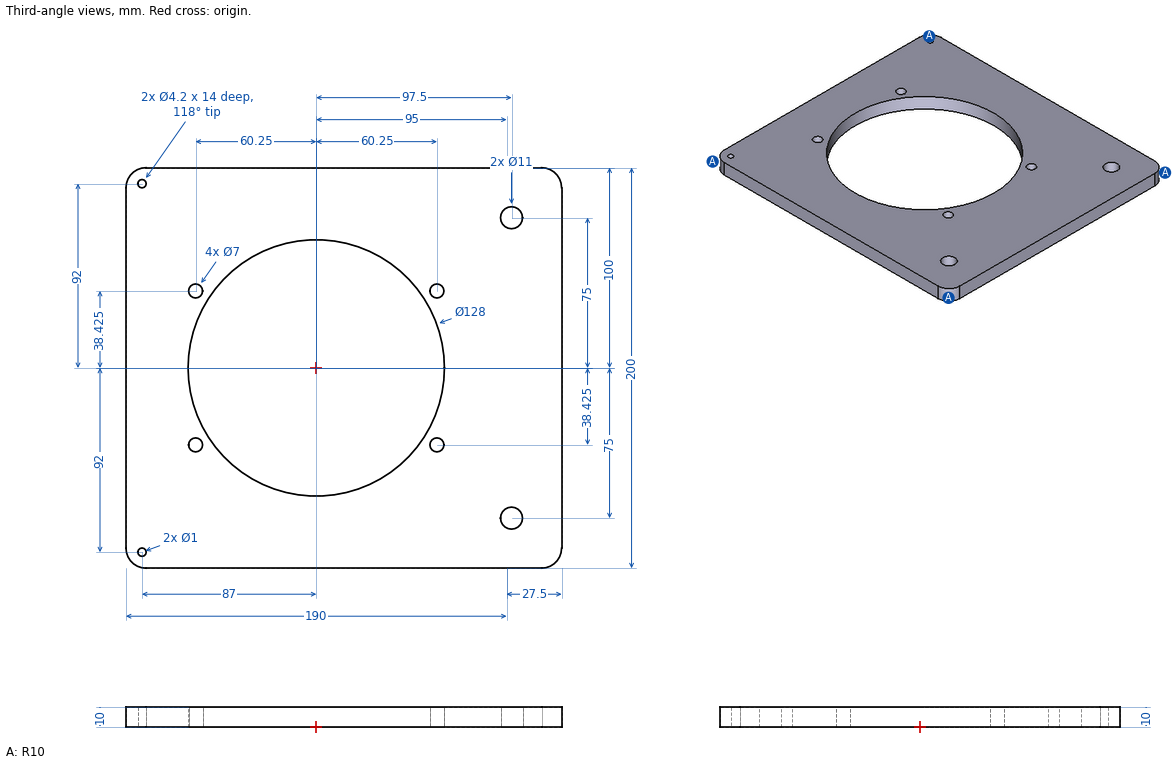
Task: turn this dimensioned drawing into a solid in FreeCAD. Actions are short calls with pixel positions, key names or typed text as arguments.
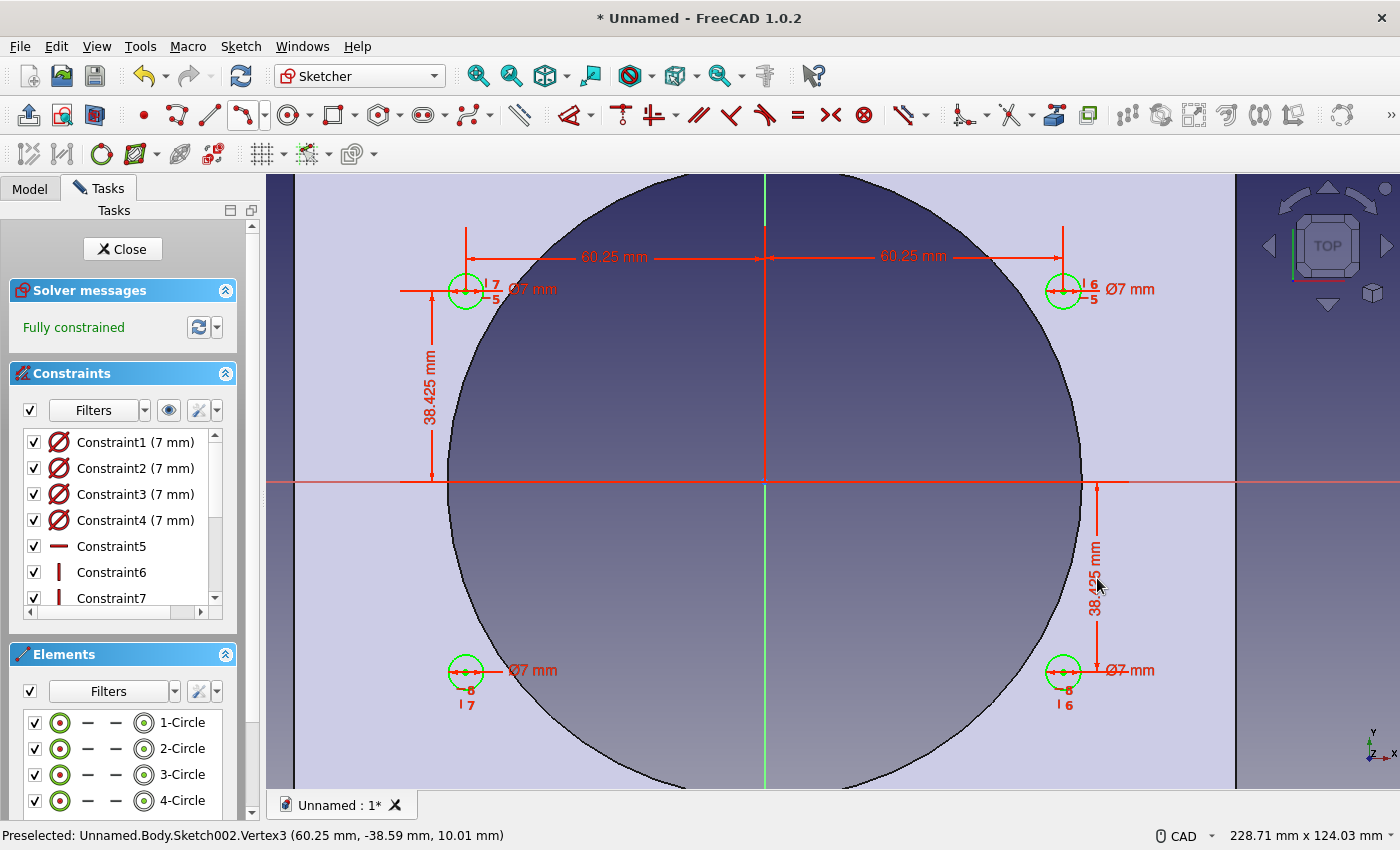
click(123, 249)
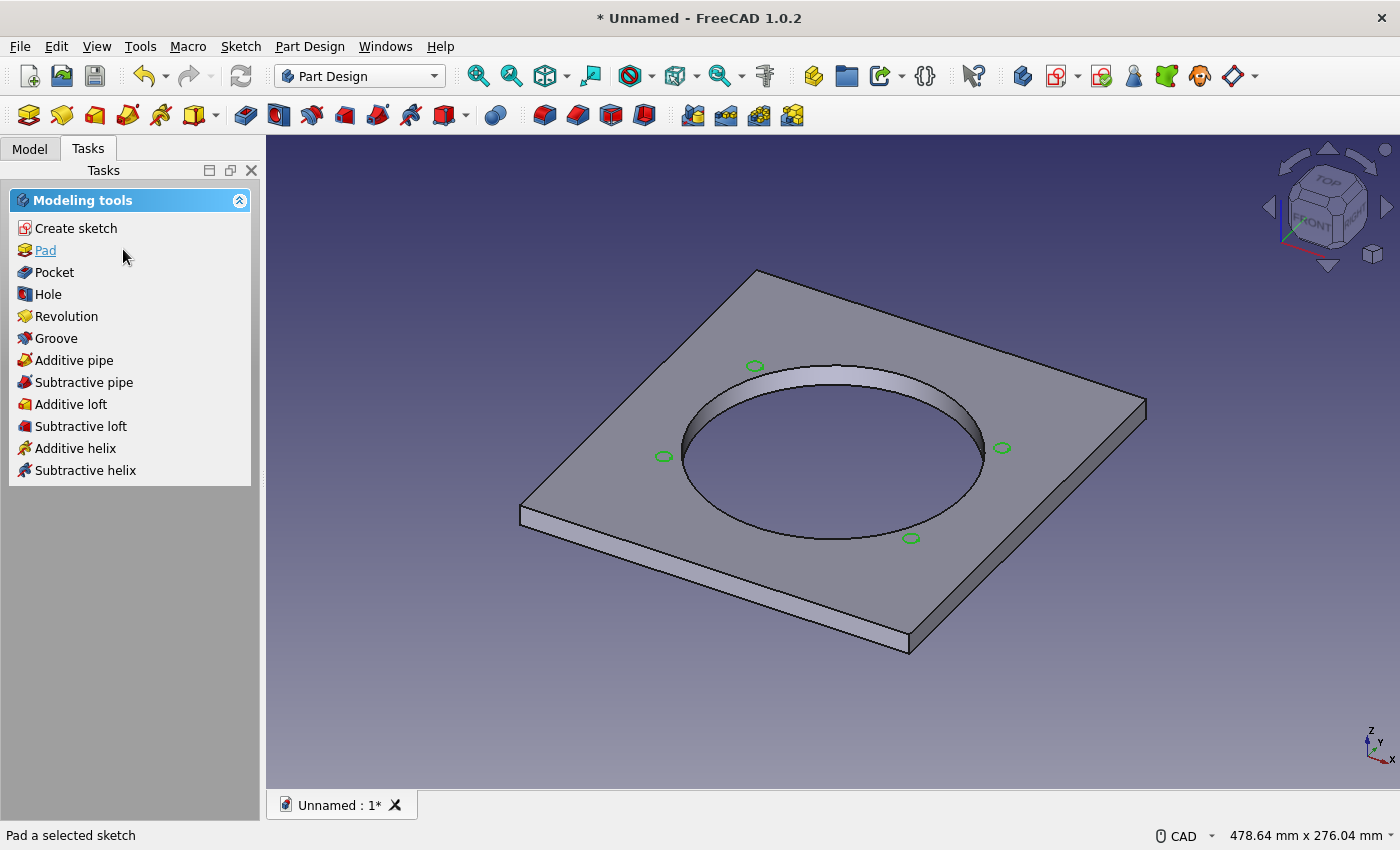
click(246, 116)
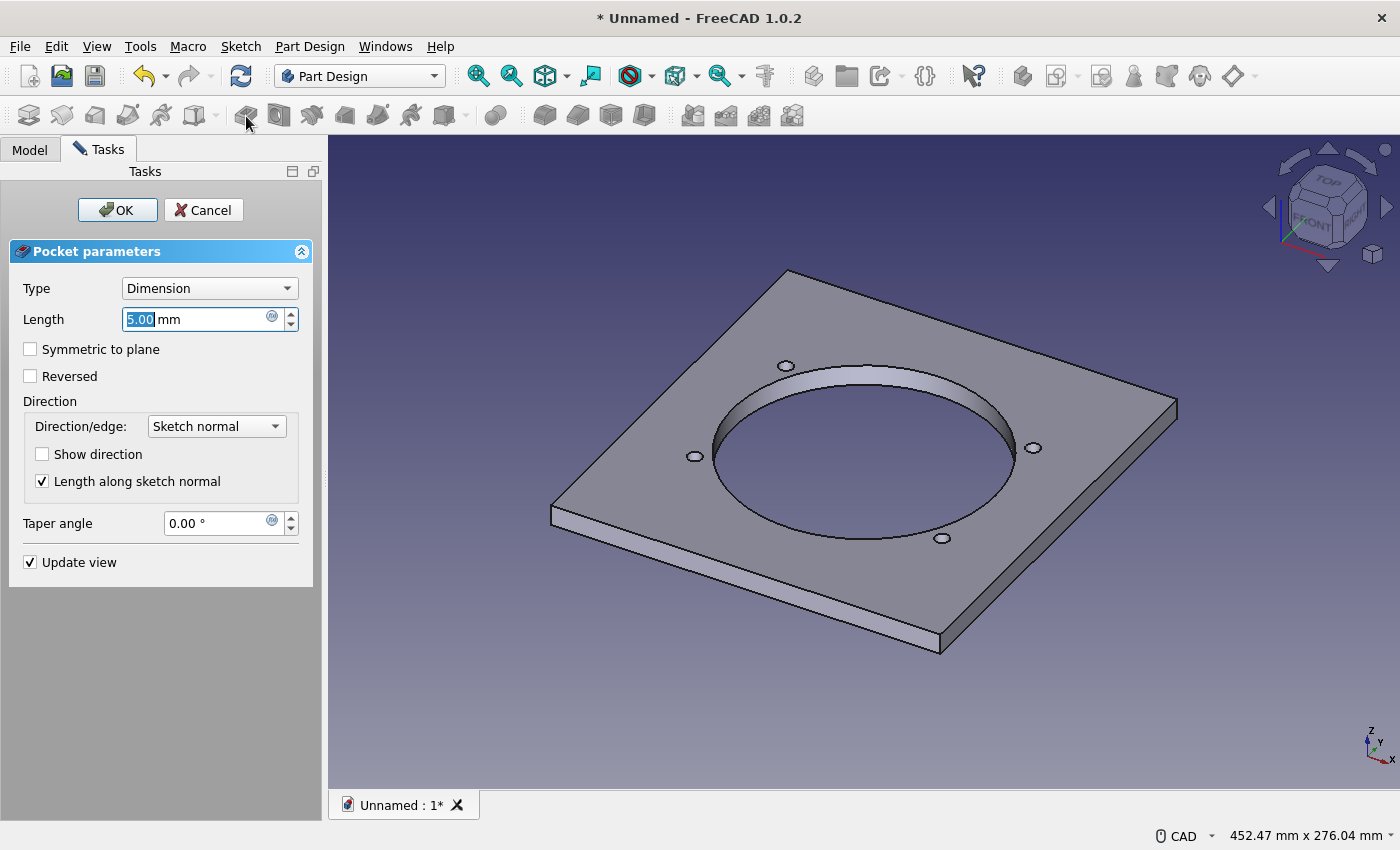
text(10)
key(Tab)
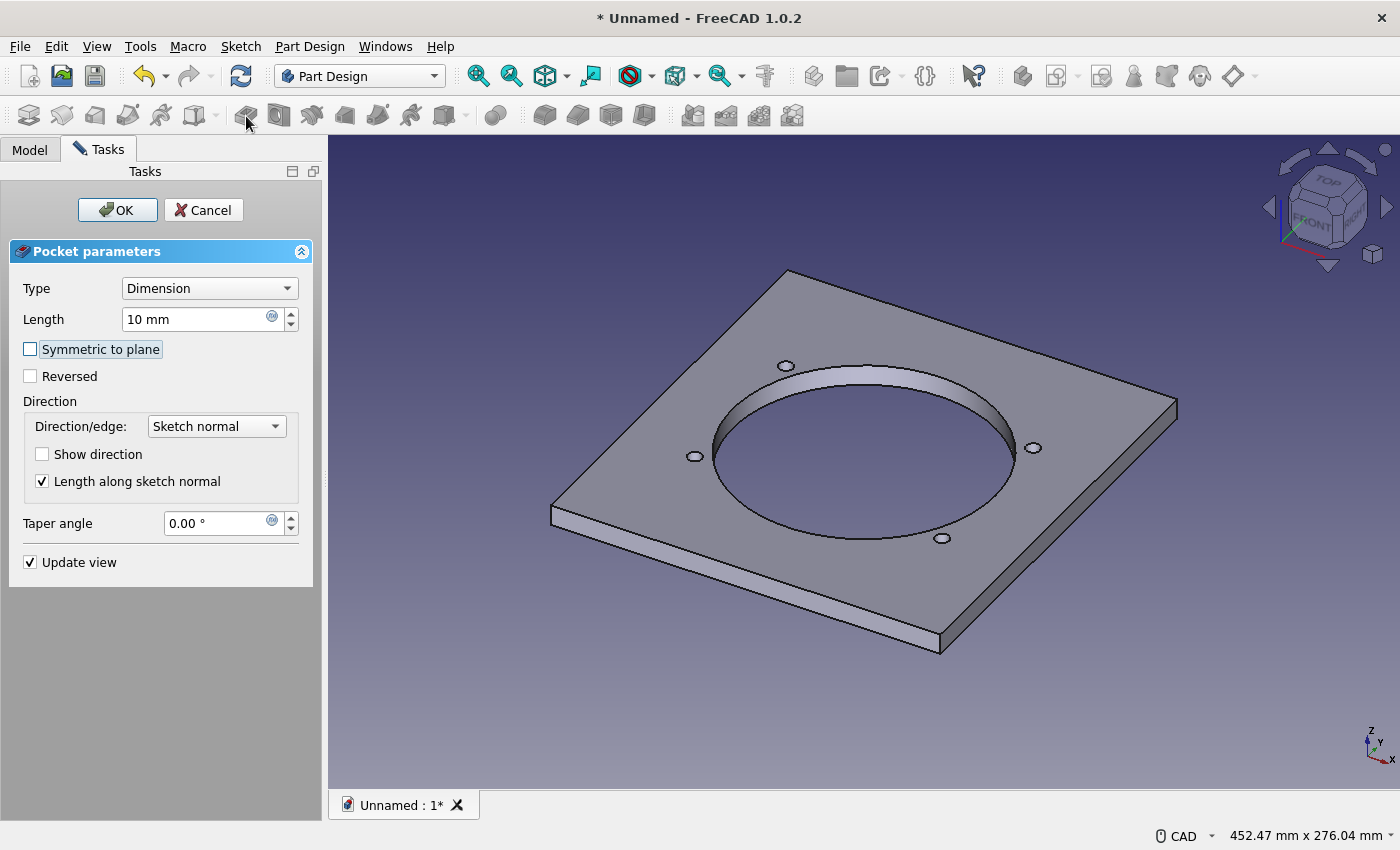
click(118, 210)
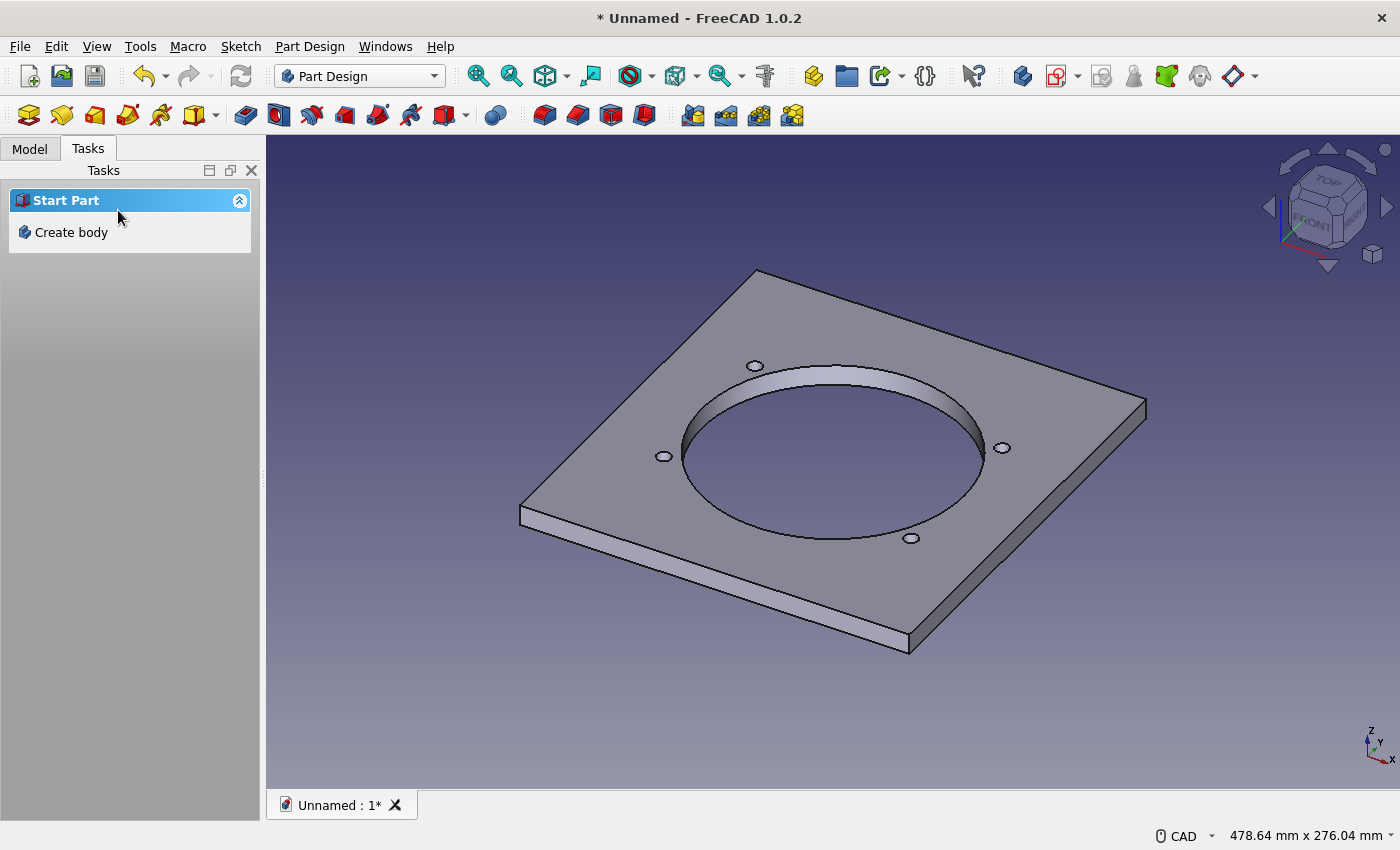
click(654, 482)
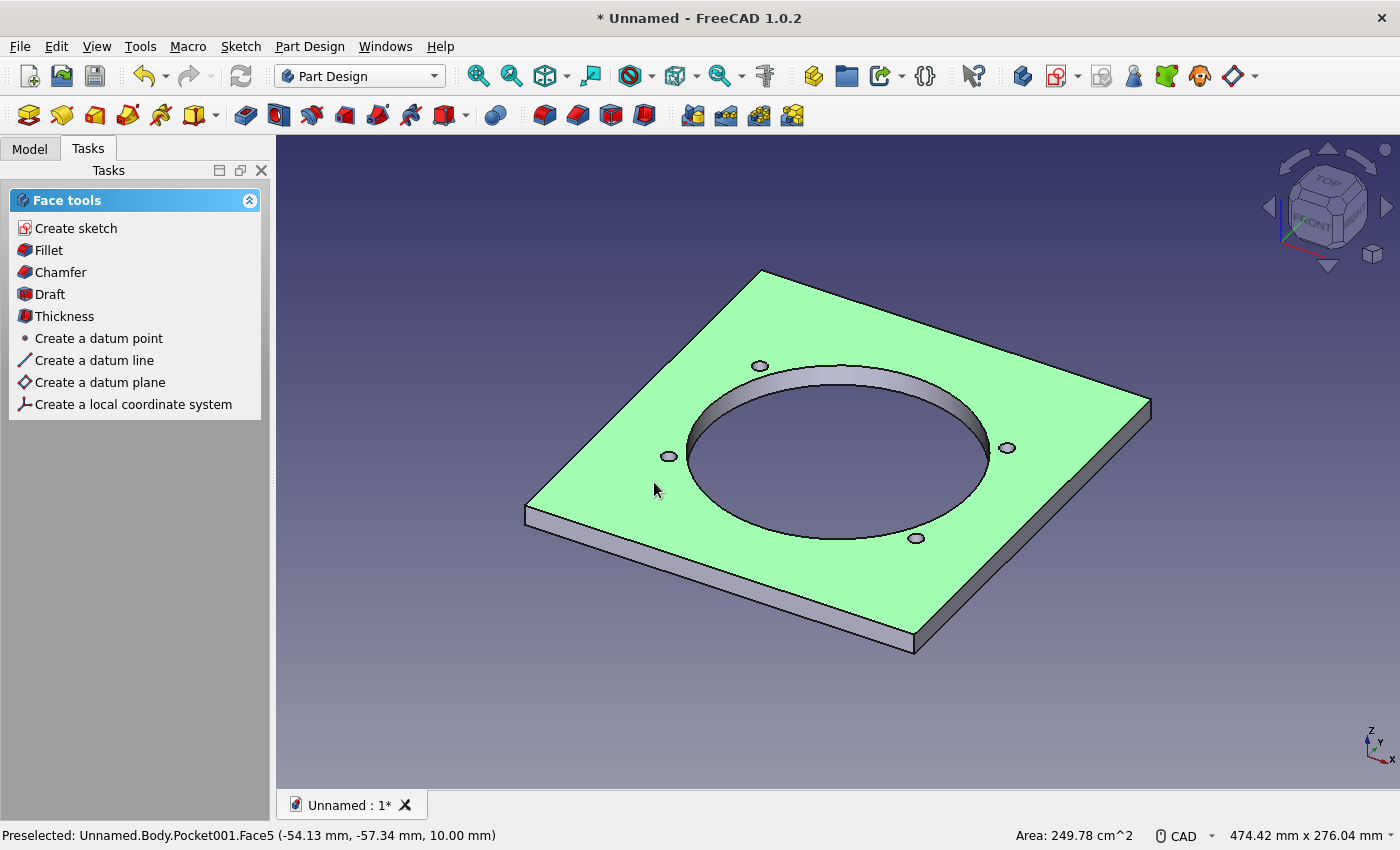
click(1056, 76)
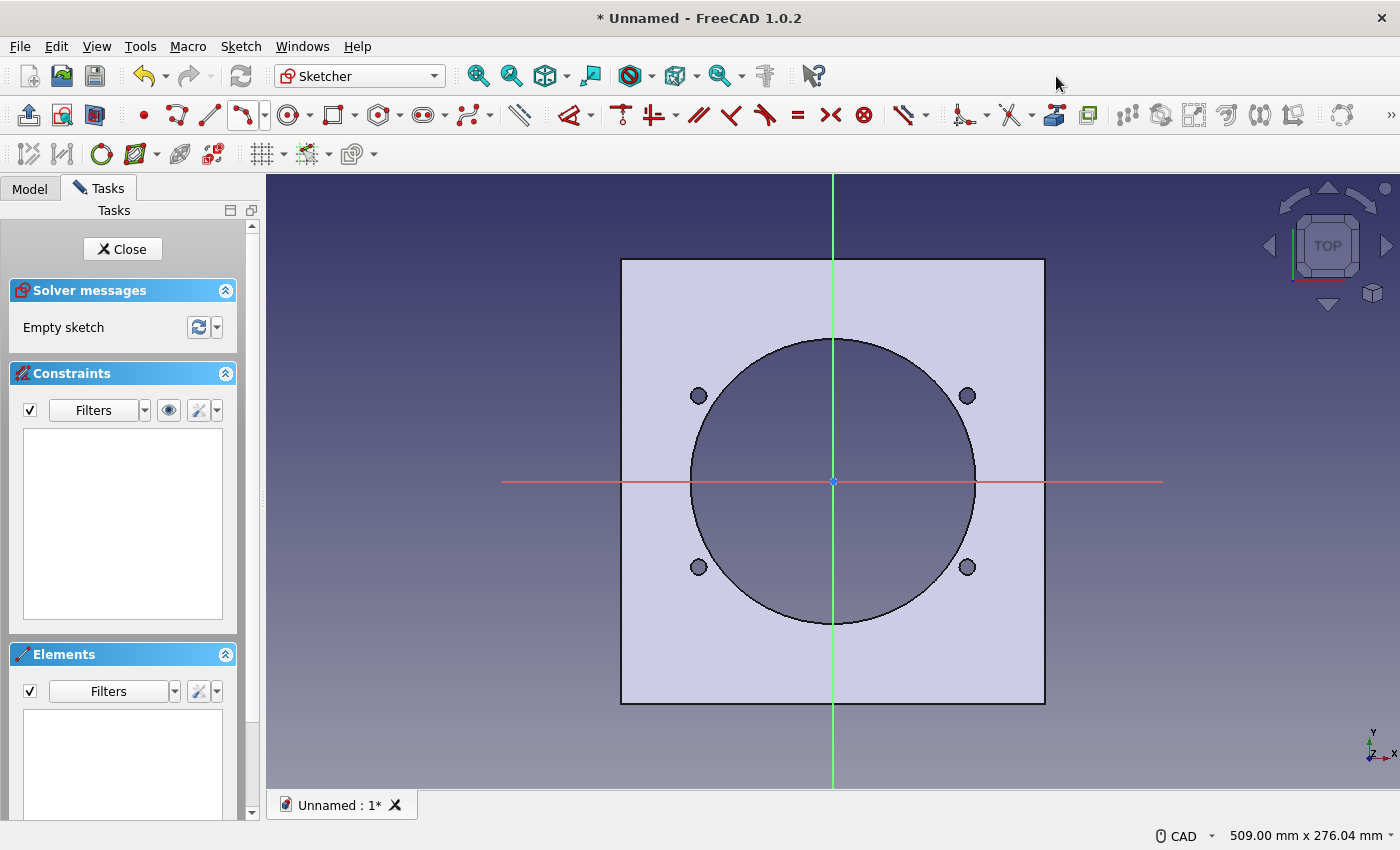
click(332, 116)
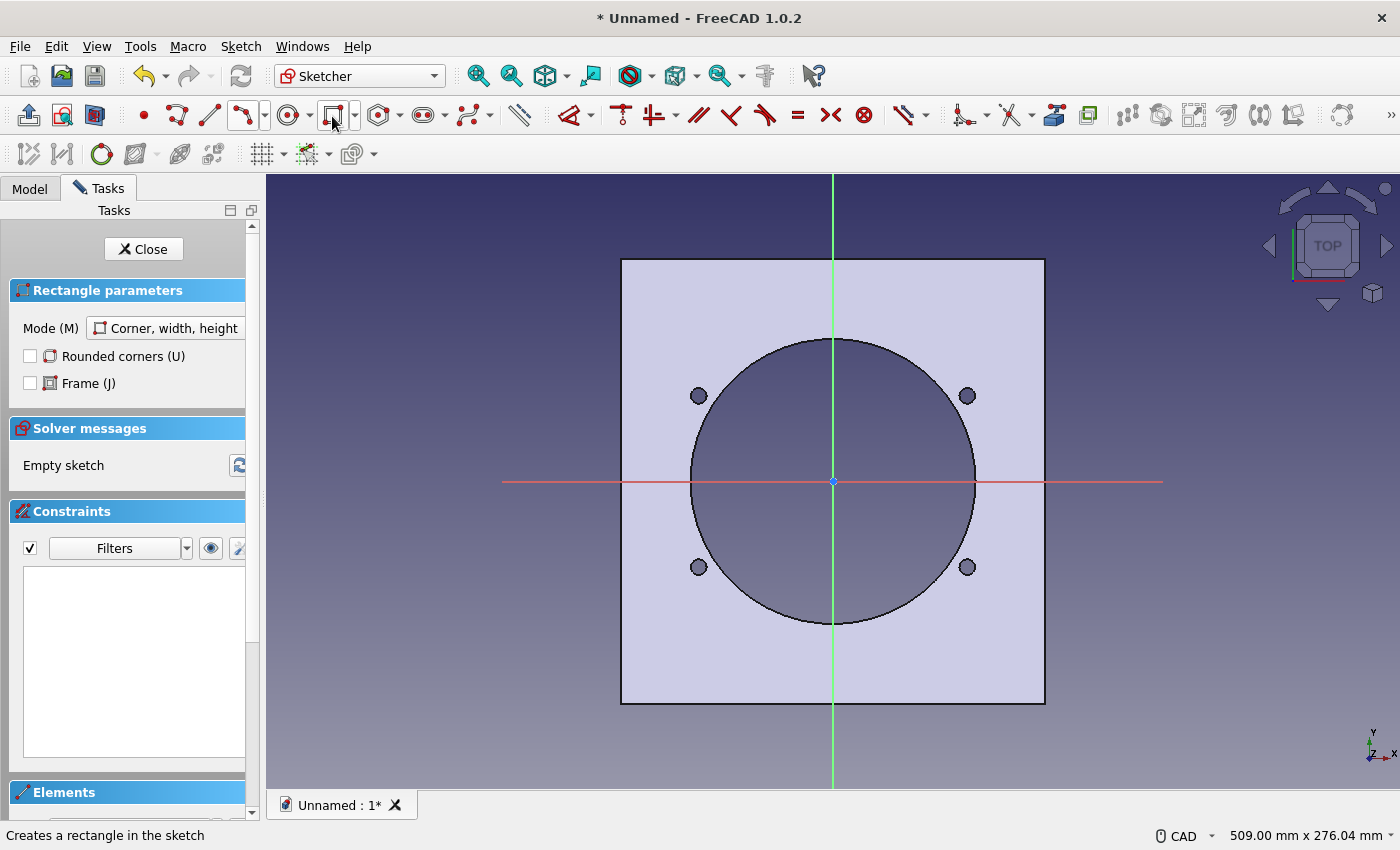
click(1045, 259)
move(1106, 704)